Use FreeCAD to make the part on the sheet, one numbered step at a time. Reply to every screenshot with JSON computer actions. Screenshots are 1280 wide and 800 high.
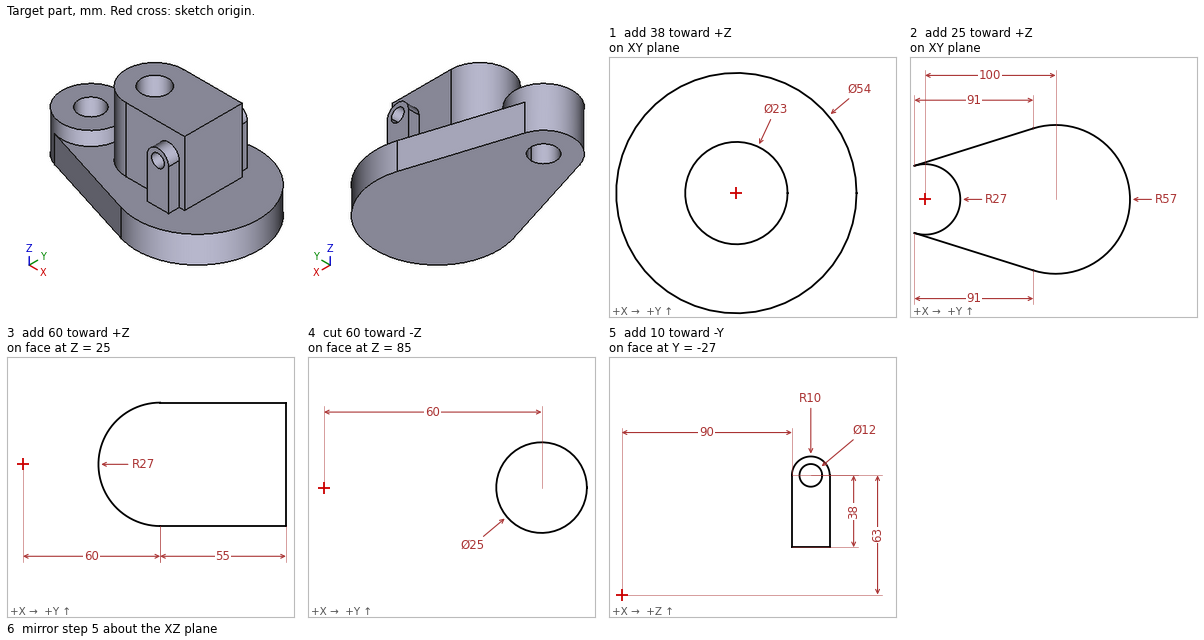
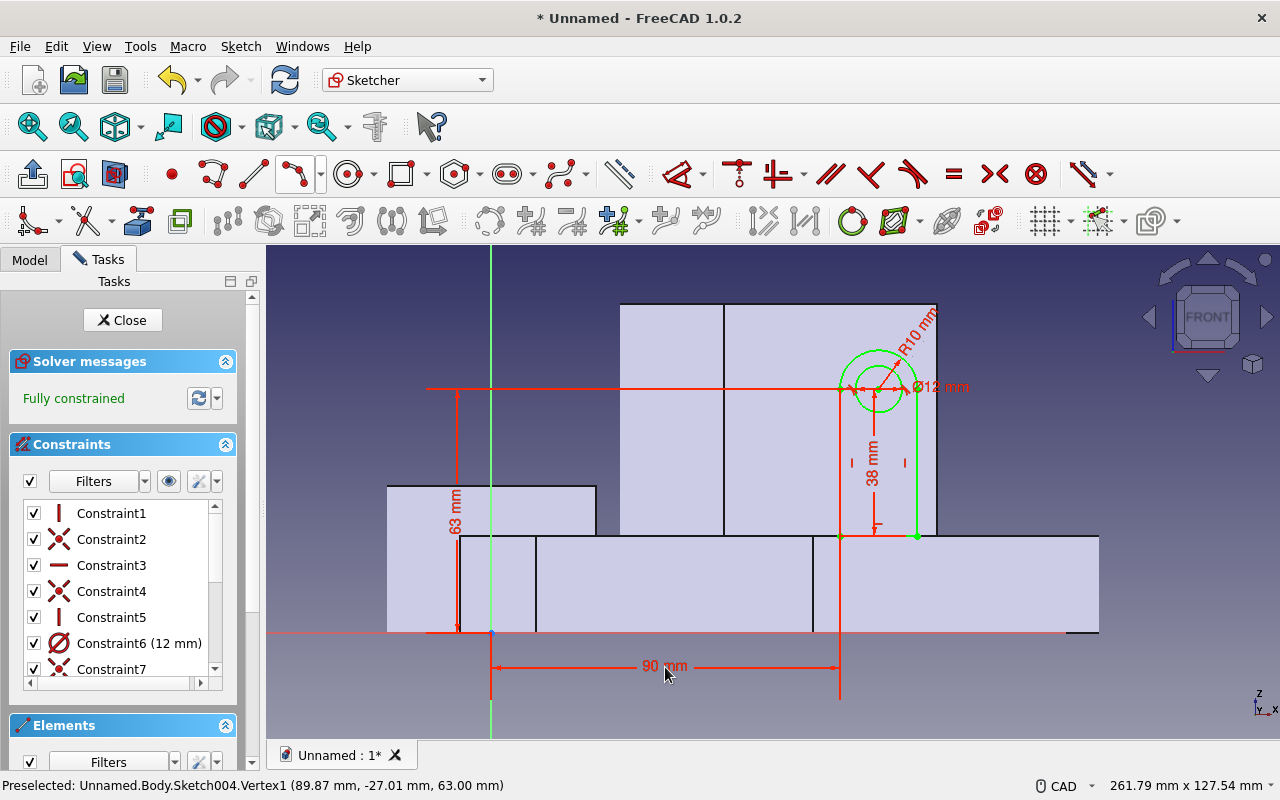
{"action": "left_click", "coordinate": [123, 320]}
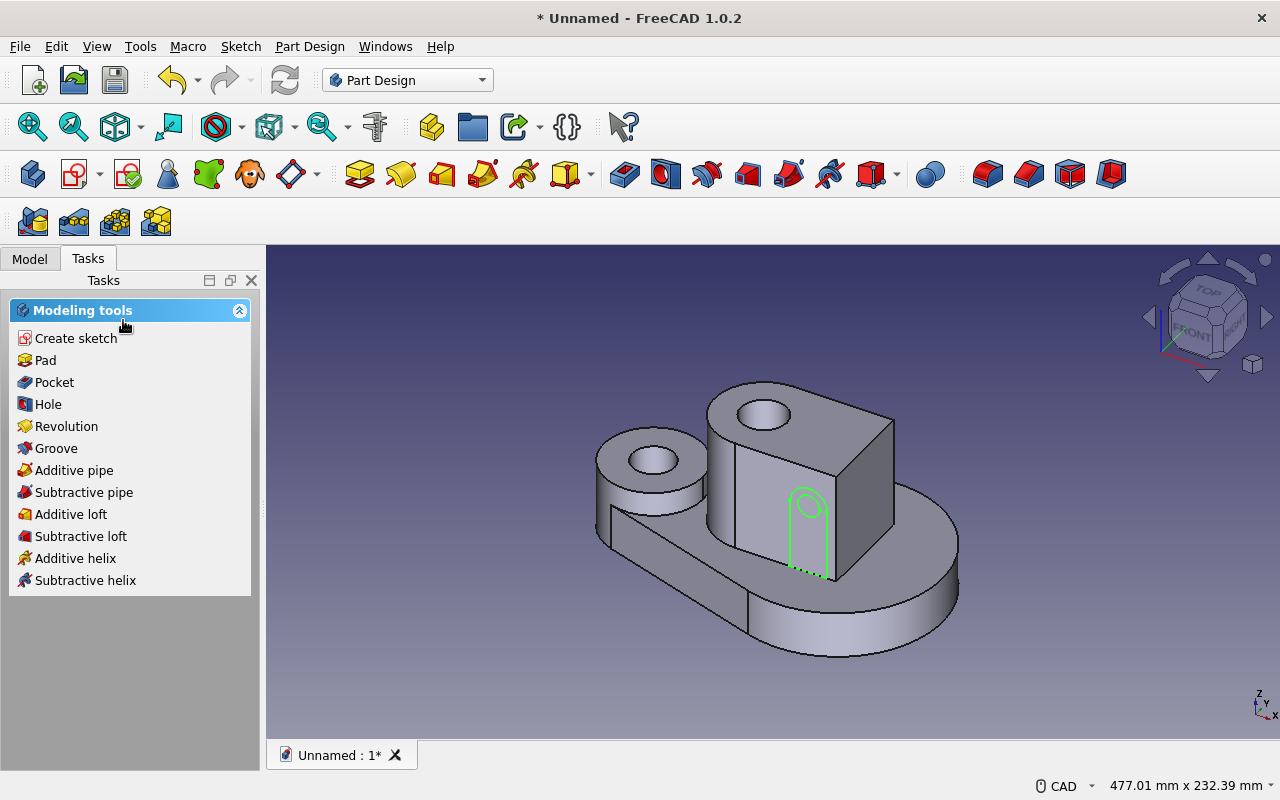
{"action": "left_click", "coordinate": [360, 174]}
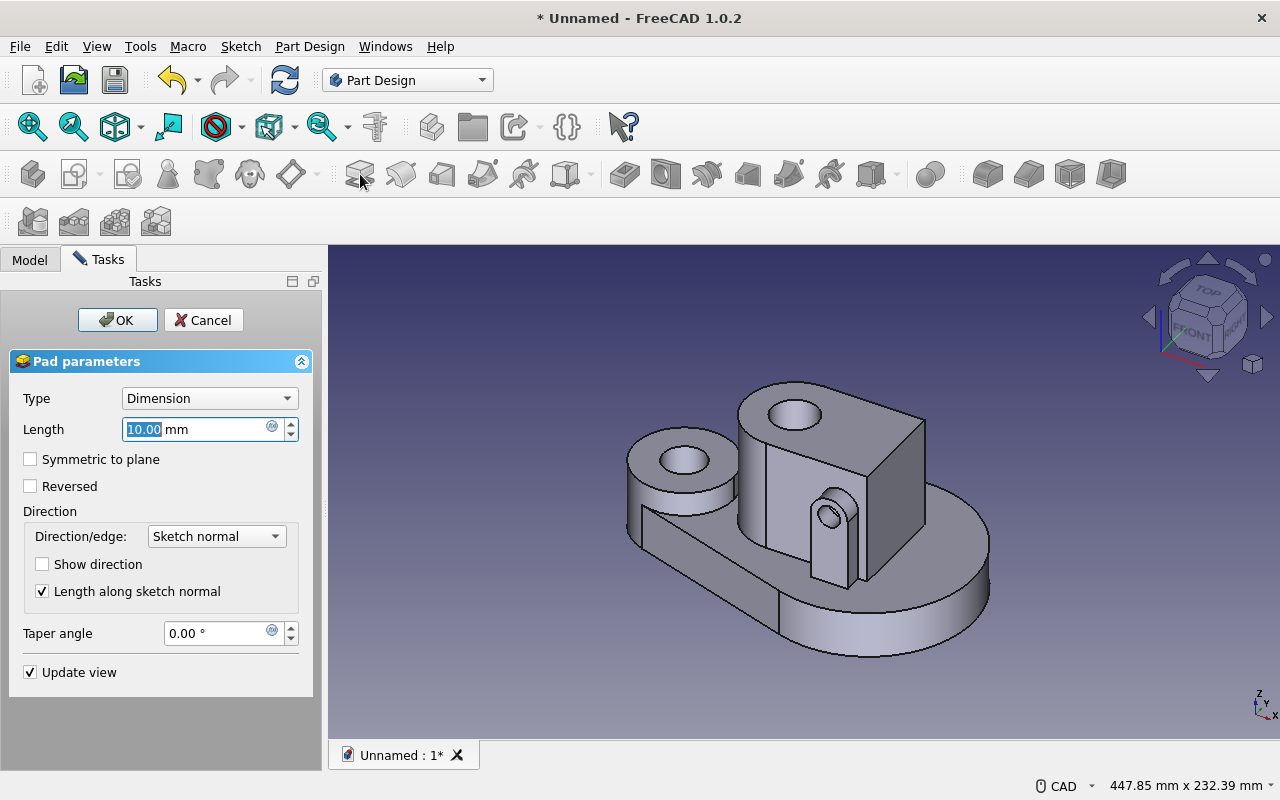
{"action": "type", "text": "10"}
{"action": "key", "text": "Tab"}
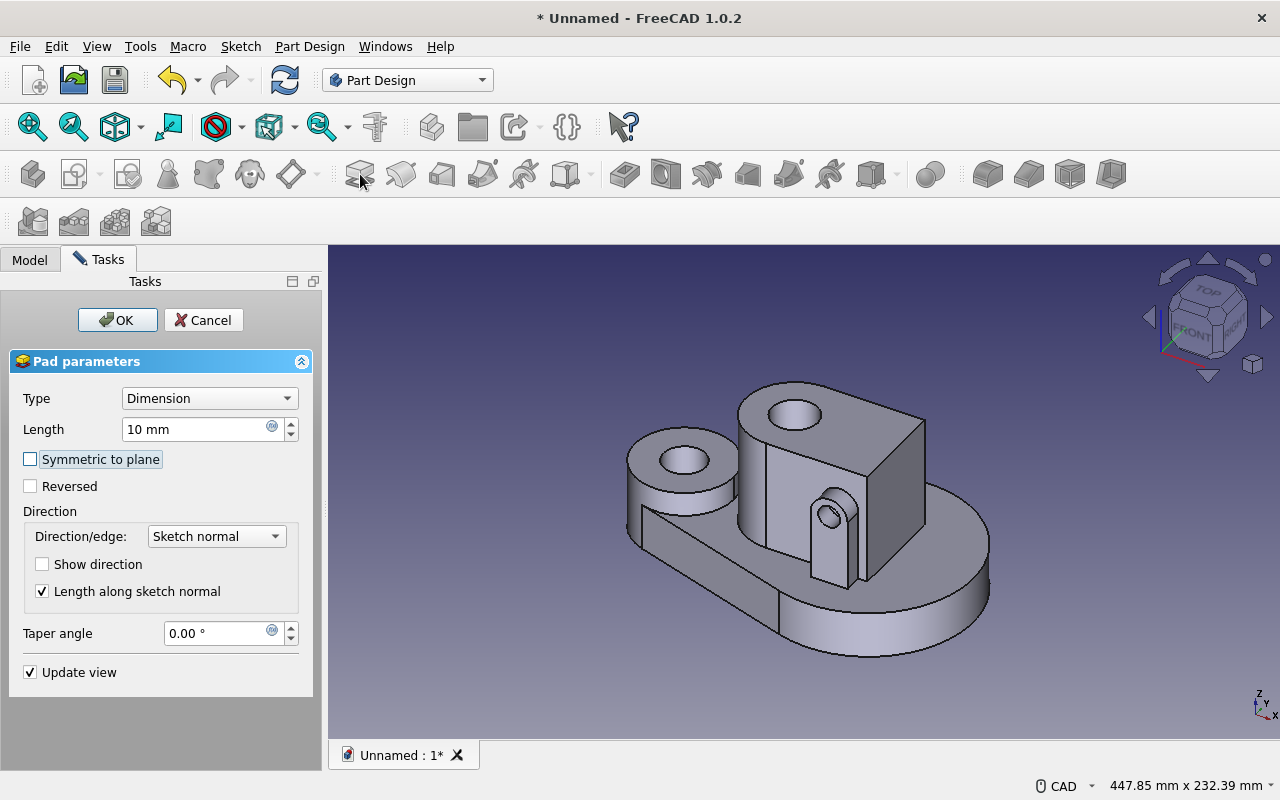
{"action": "left_click", "coordinate": [118, 320]}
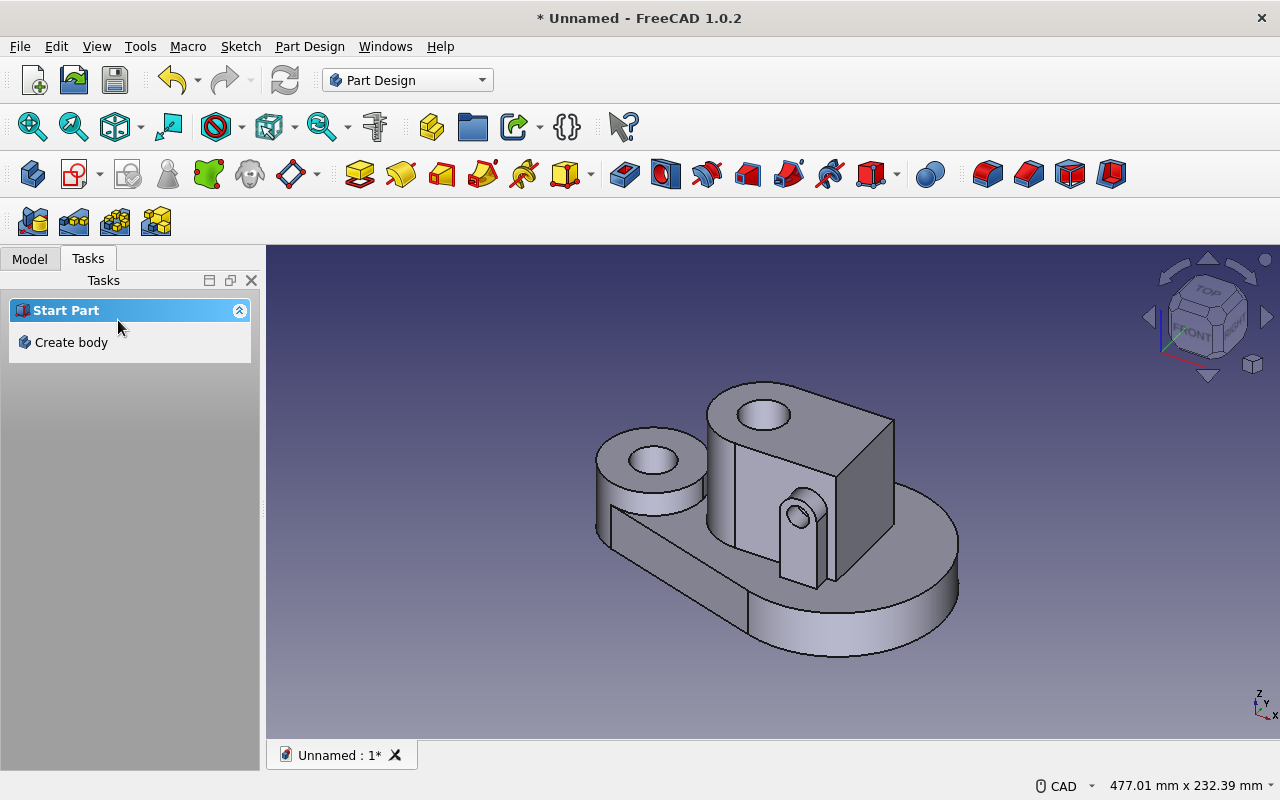
{"action": "left_click", "coordinate": [30, 258]}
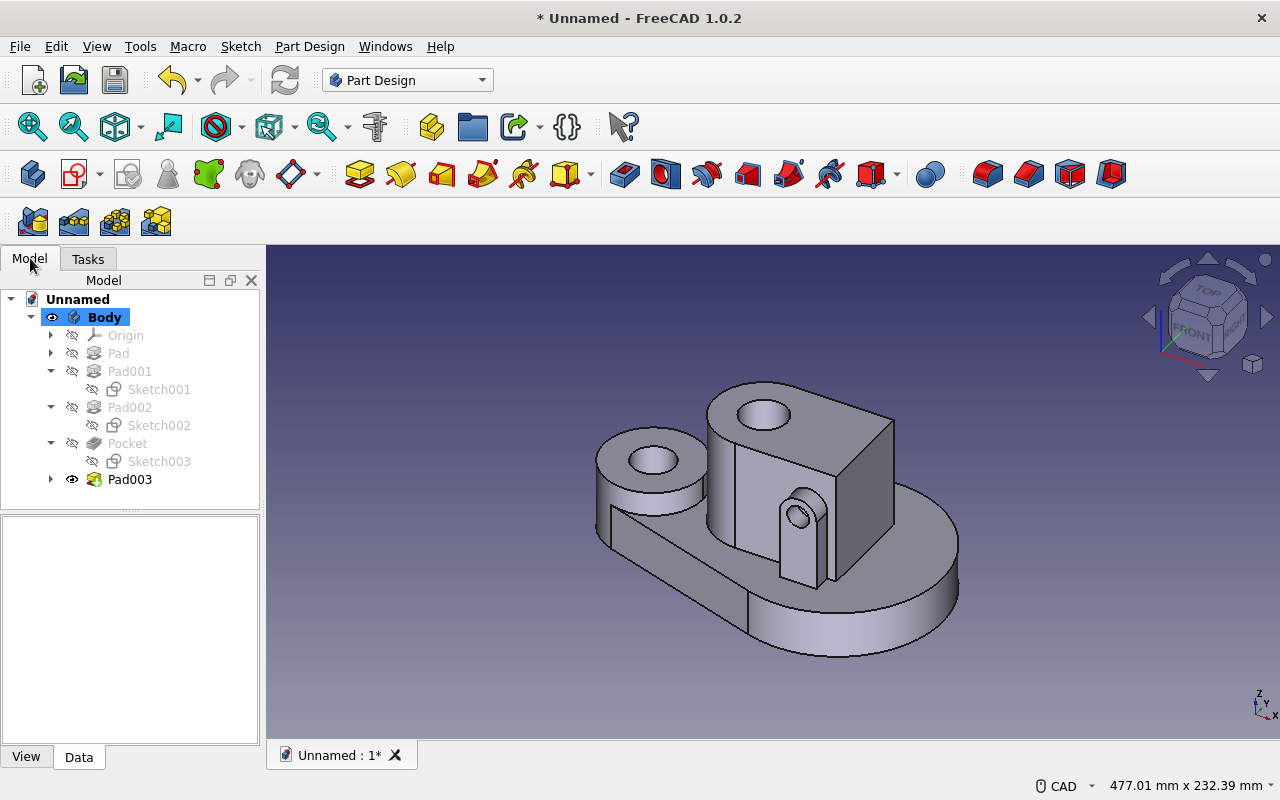
{"action": "left_click", "coordinate": [117, 479]}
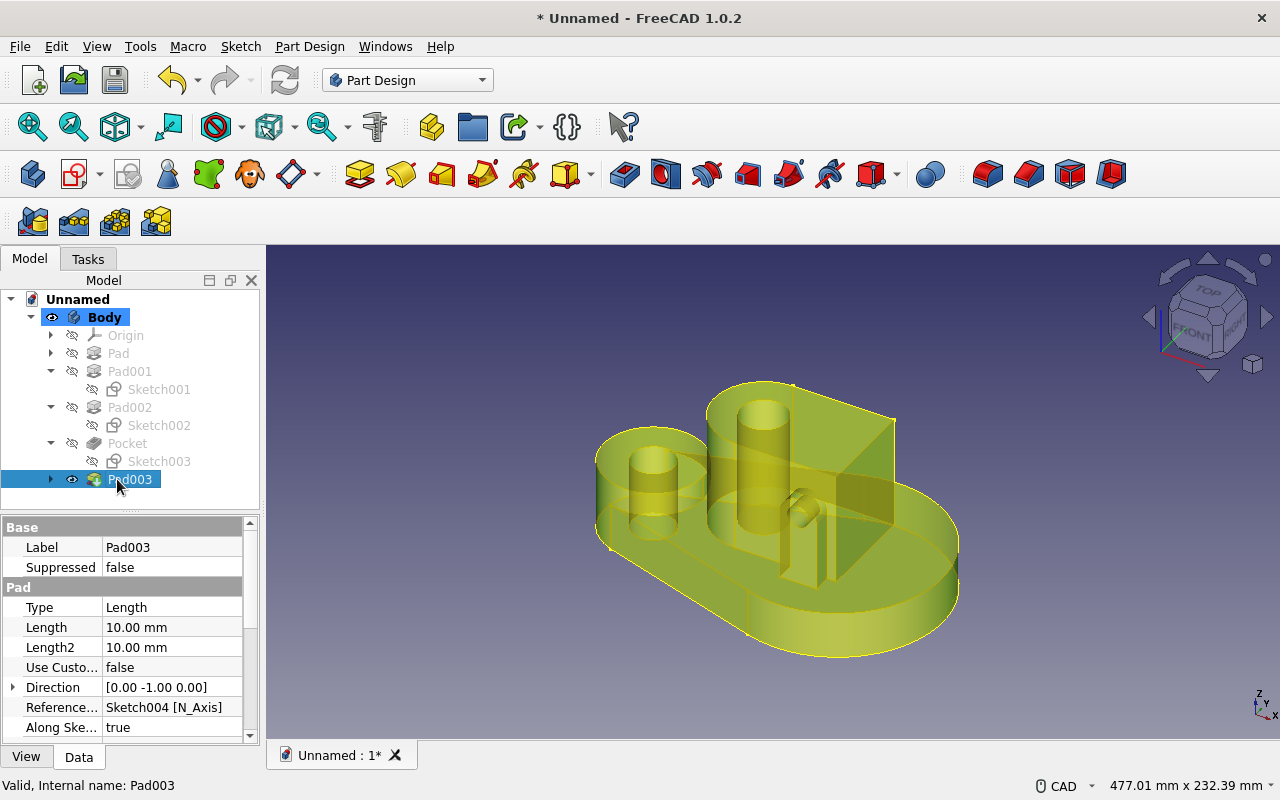
{"action": "left_click", "coordinate": [33, 222]}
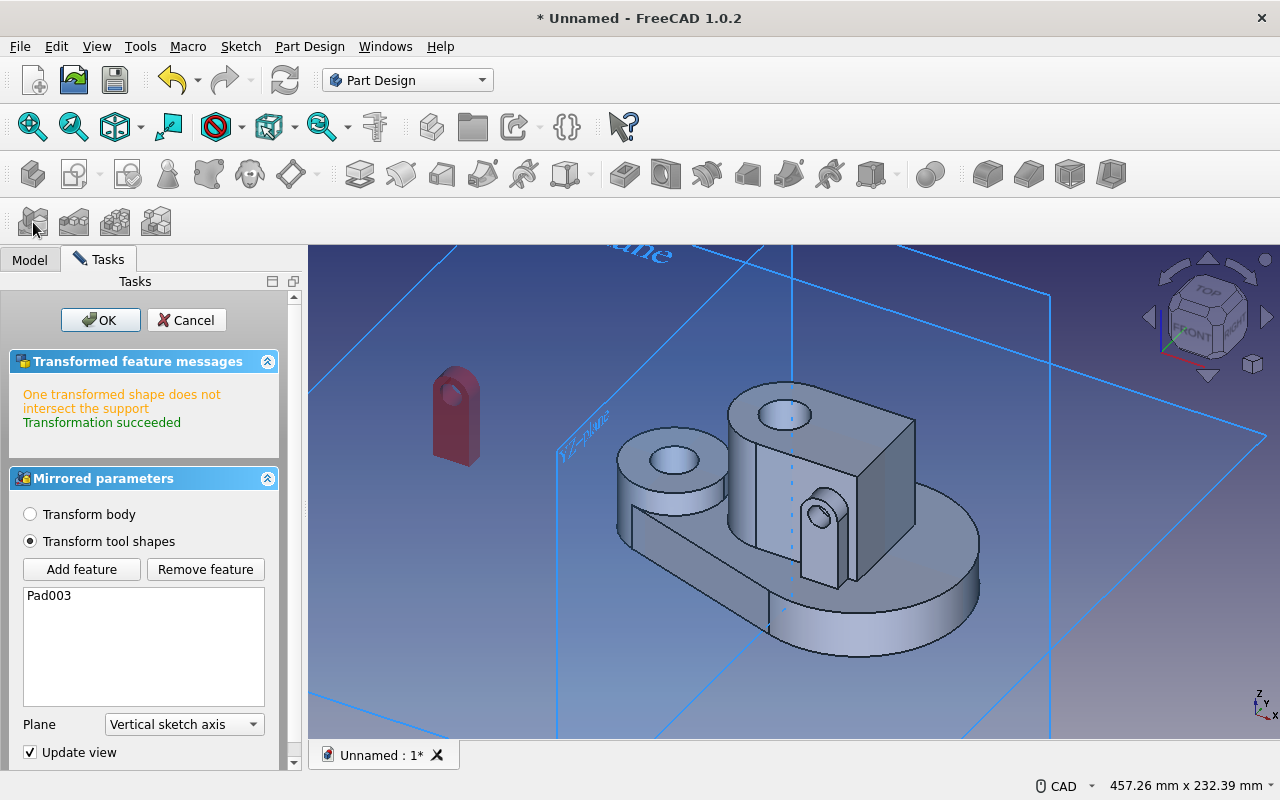
{"action": "left_click", "coordinate": [185, 724]}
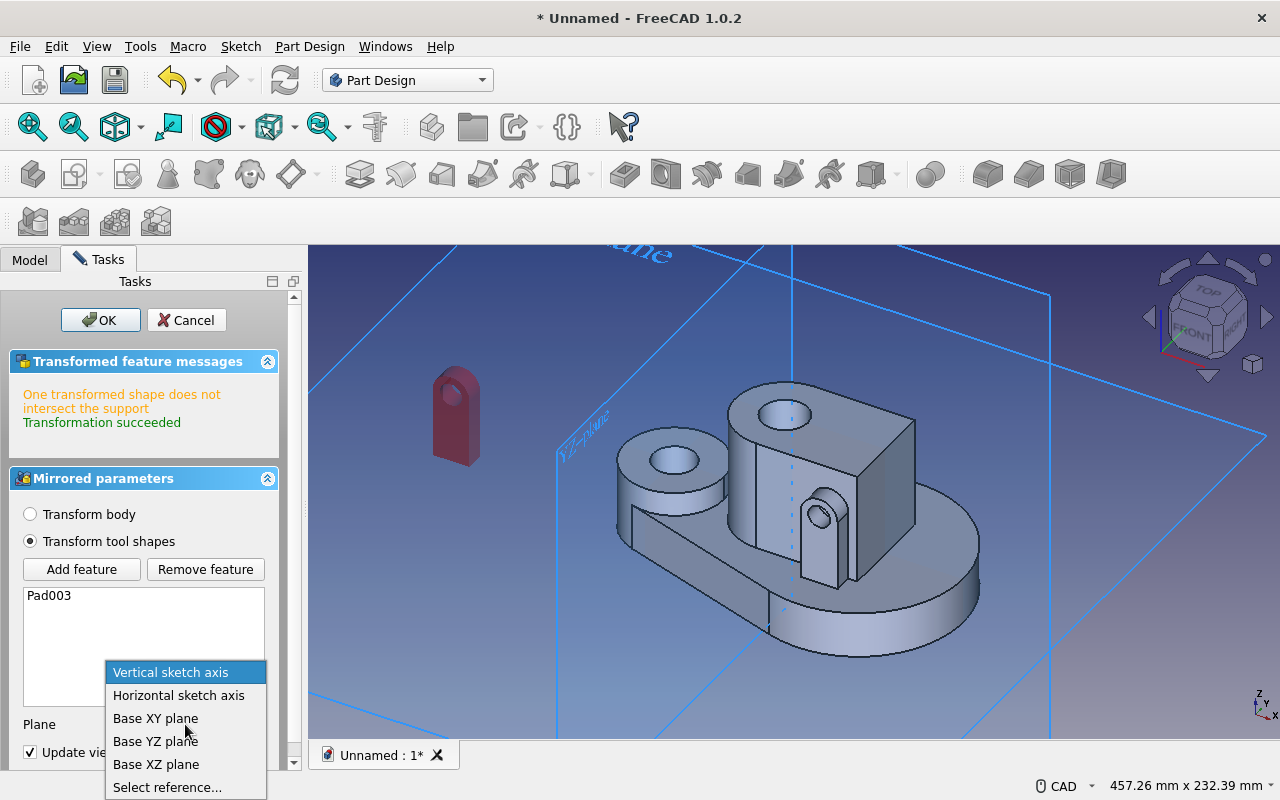
{"action": "left_click", "coordinate": [184, 764]}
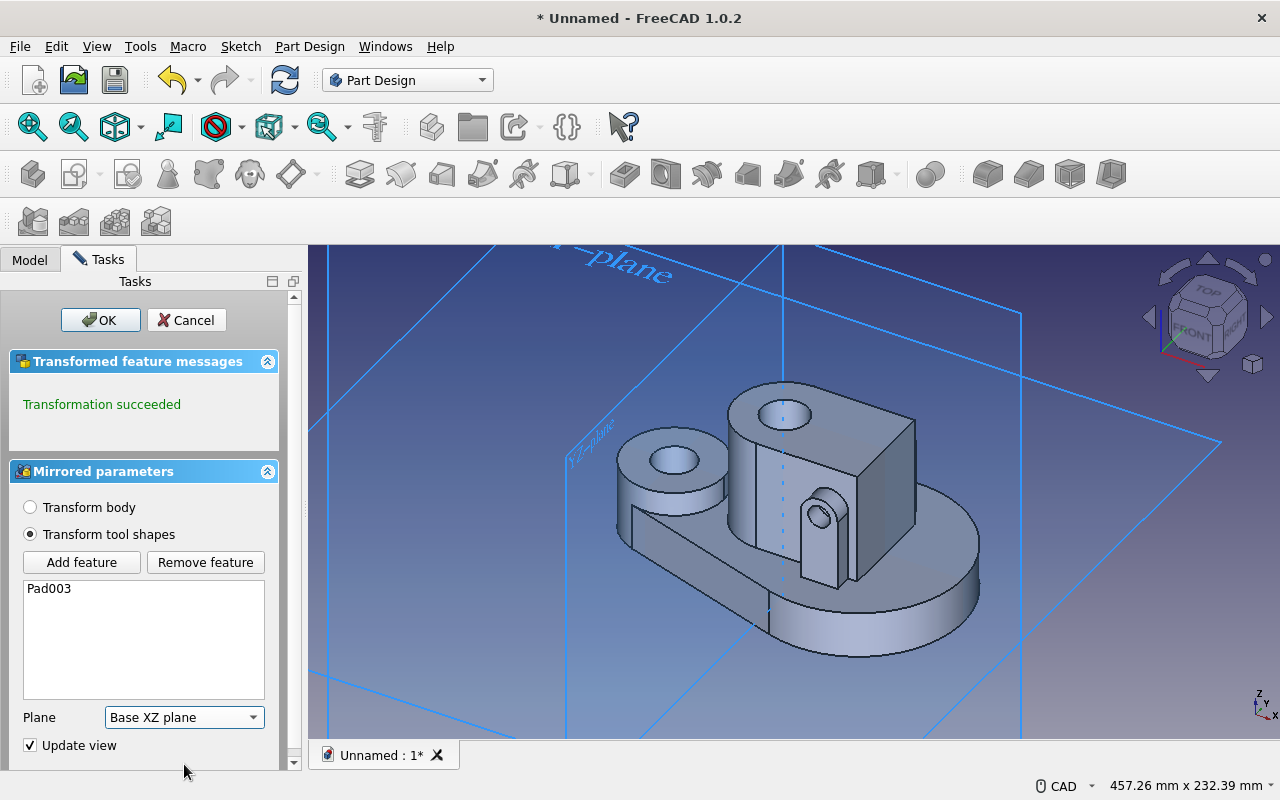
{"action": "left_click", "coordinate": [101, 320]}